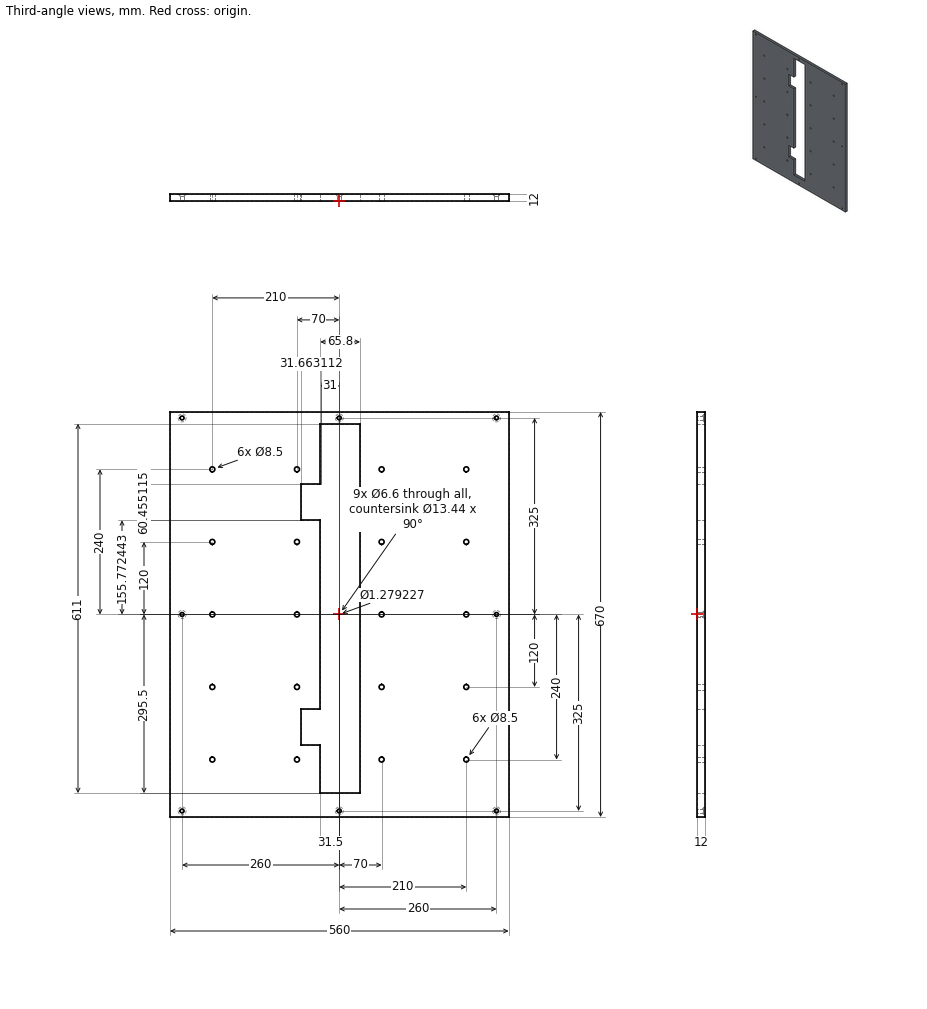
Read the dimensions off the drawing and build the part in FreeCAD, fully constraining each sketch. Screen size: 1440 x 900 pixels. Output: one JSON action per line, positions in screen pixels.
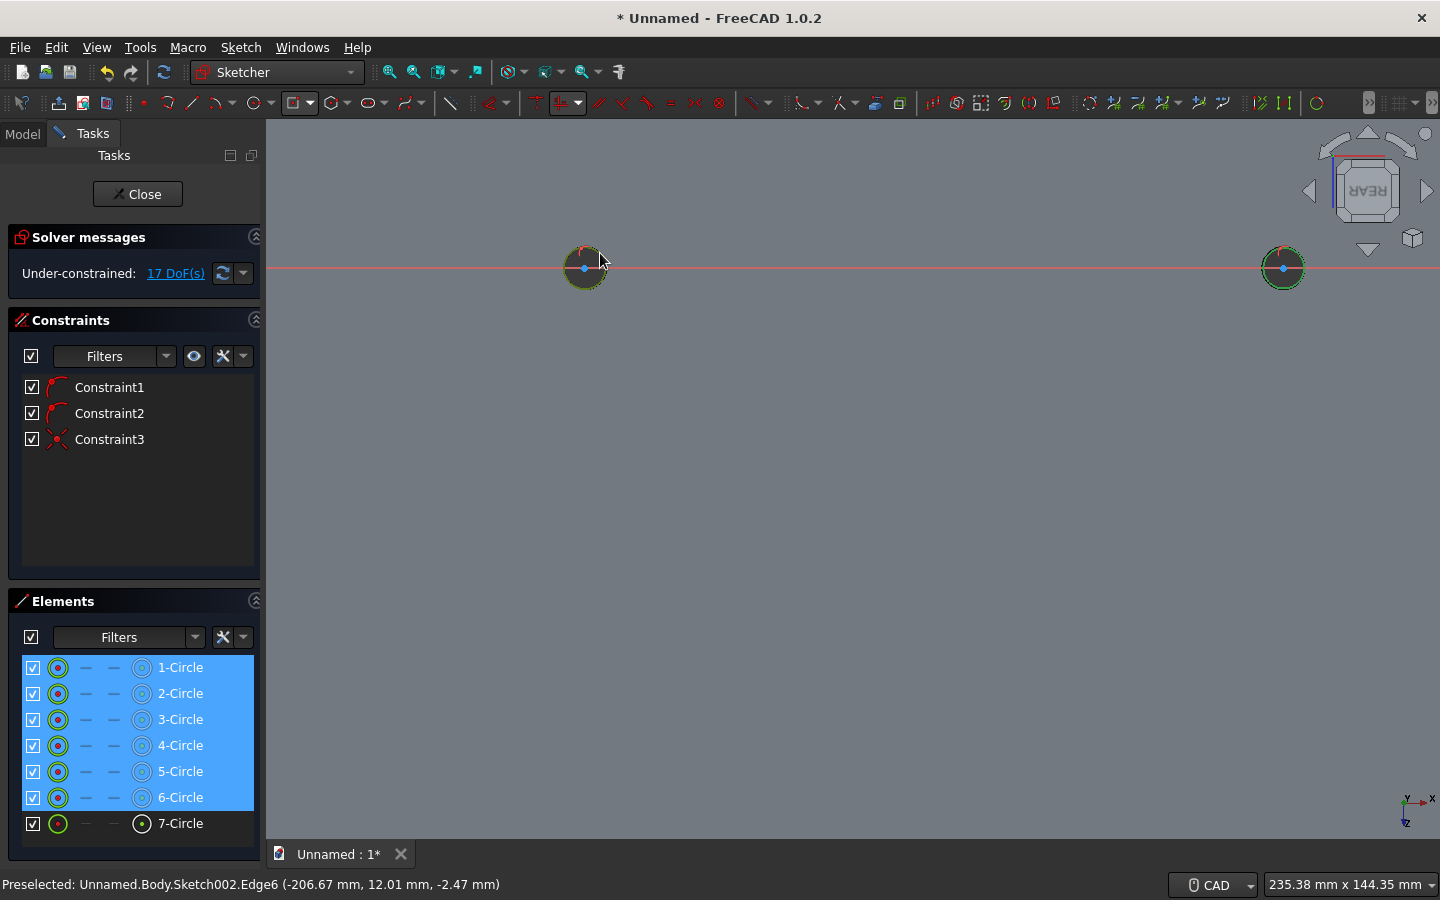
{"action": "left_click", "coordinate": [672, 104]}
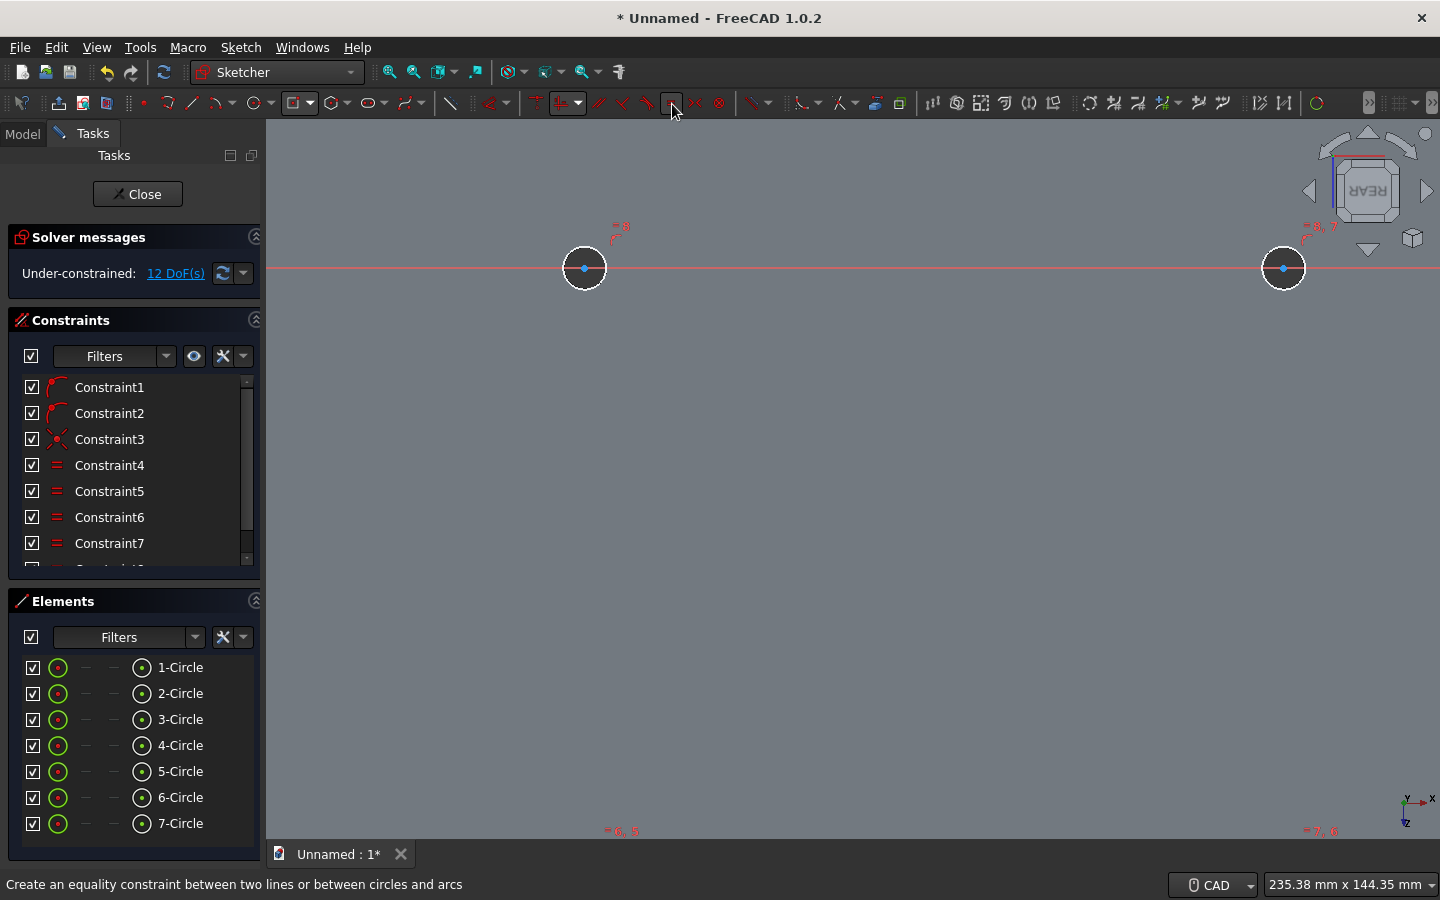
{"action": "scroll", "coordinate": [601, 253], "scroll_direction": "down", "scroll_amount": 5}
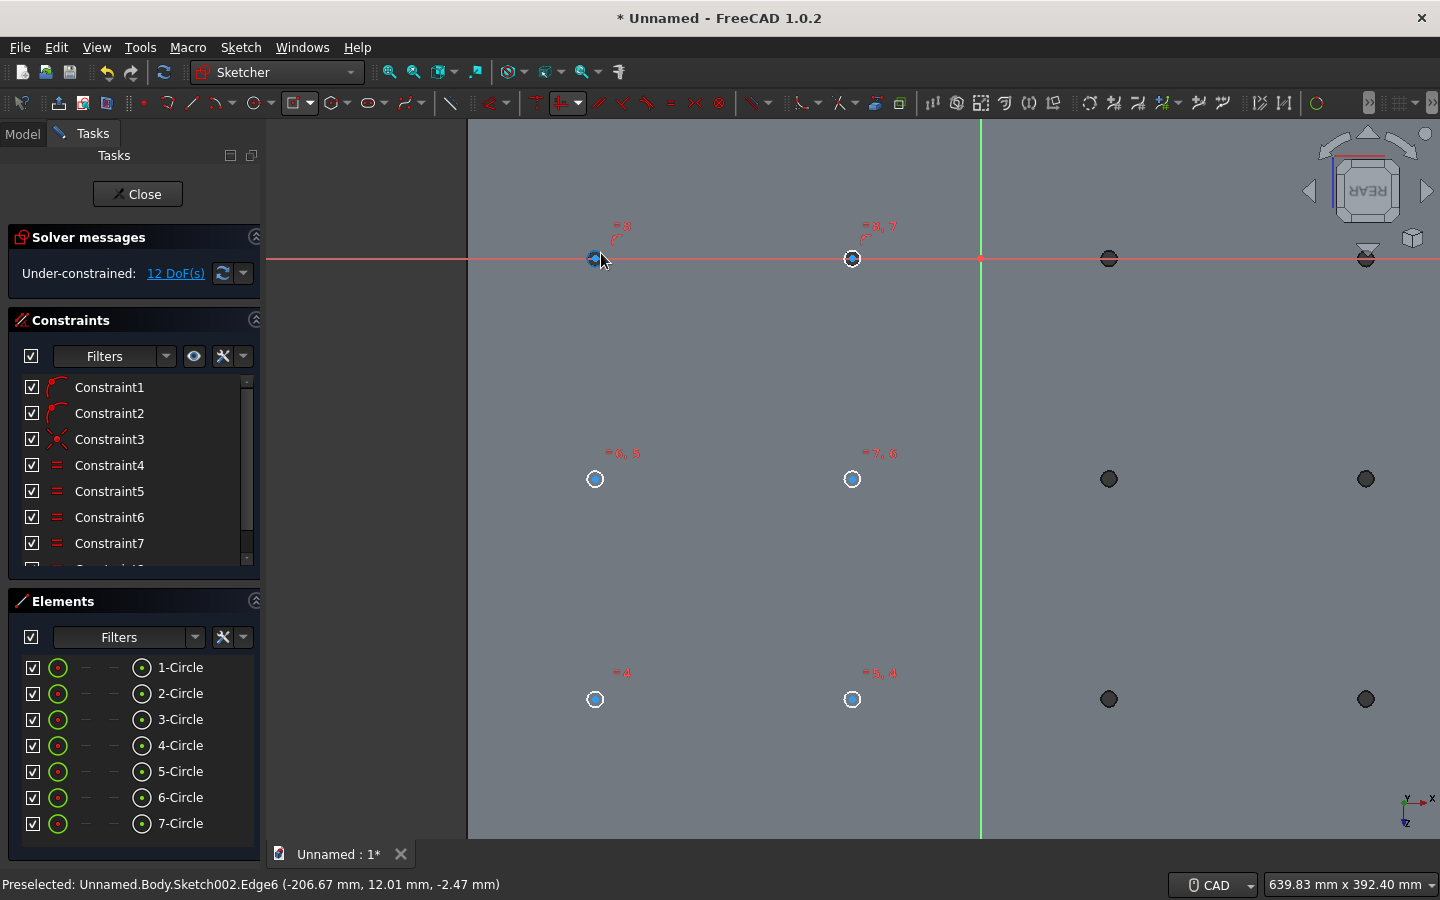
{"action": "left_click", "coordinate": [595, 699]}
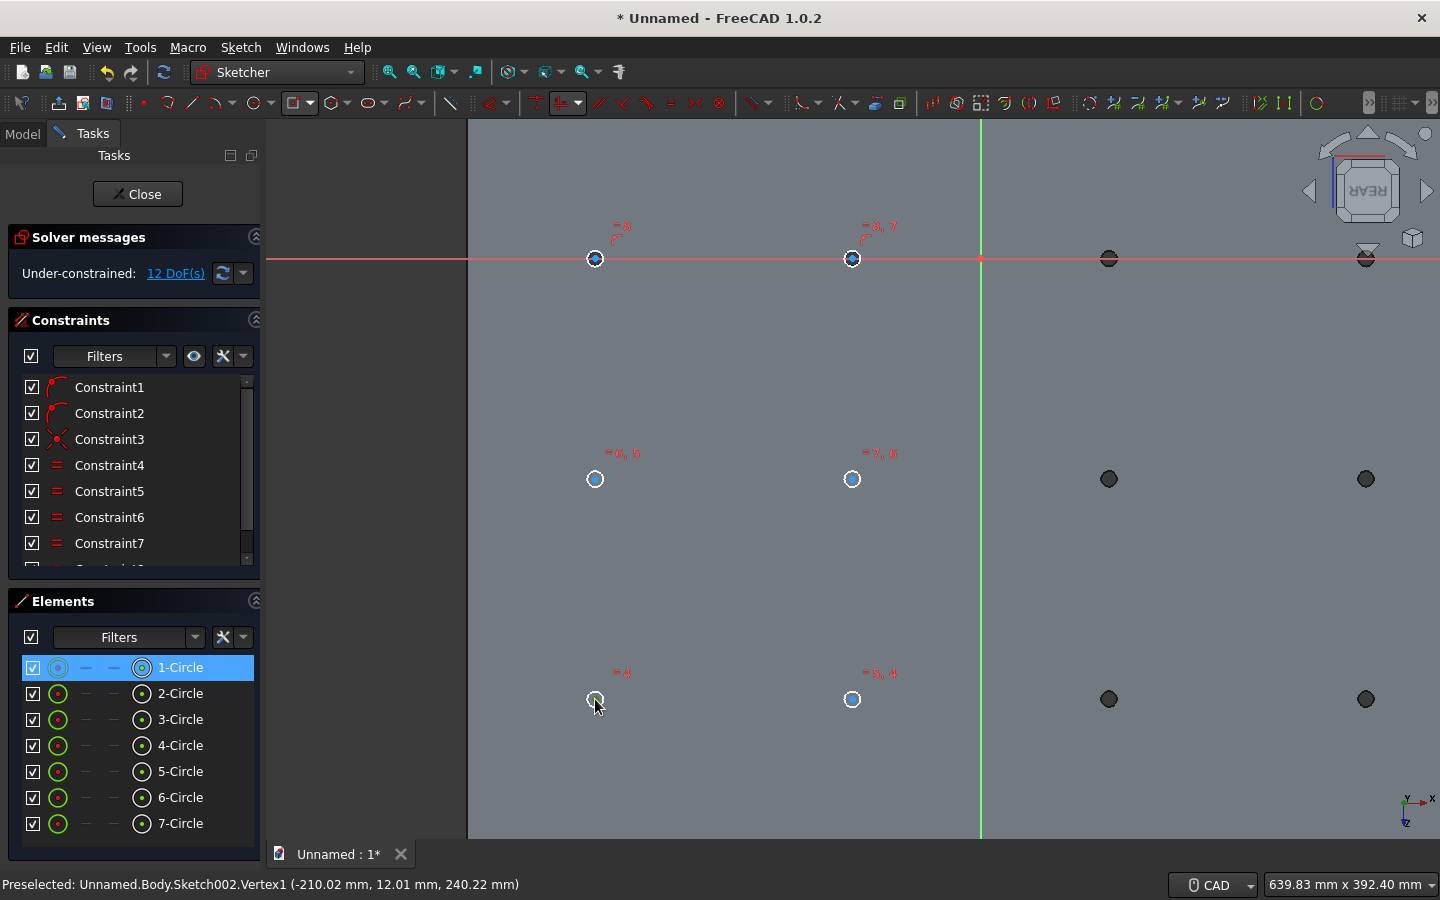
{"action": "left_click", "coordinate": [852, 699]}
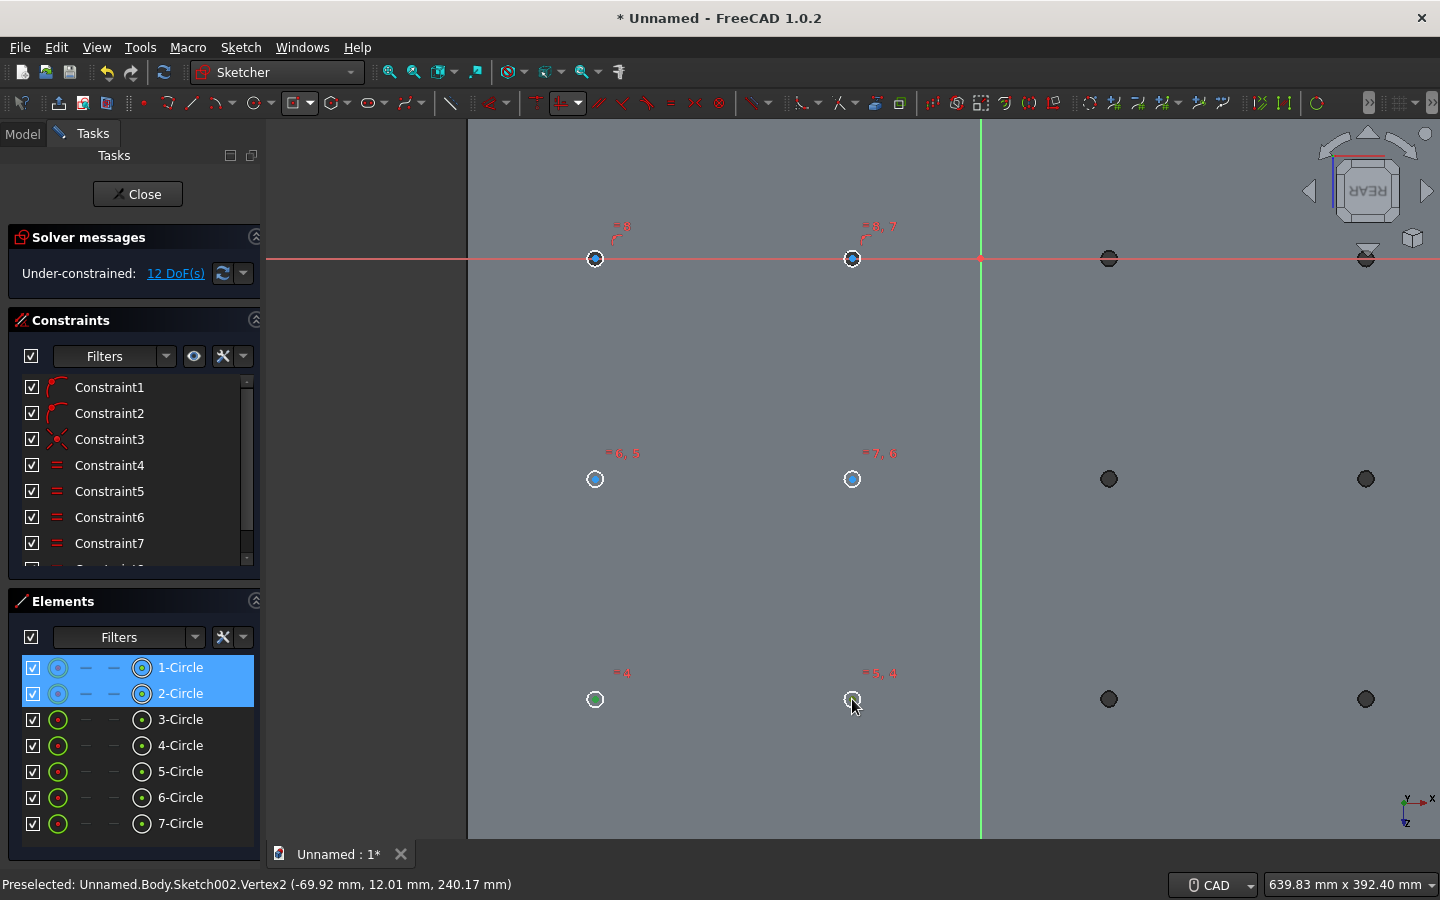
{"action": "left_click", "coordinate": [580, 104]}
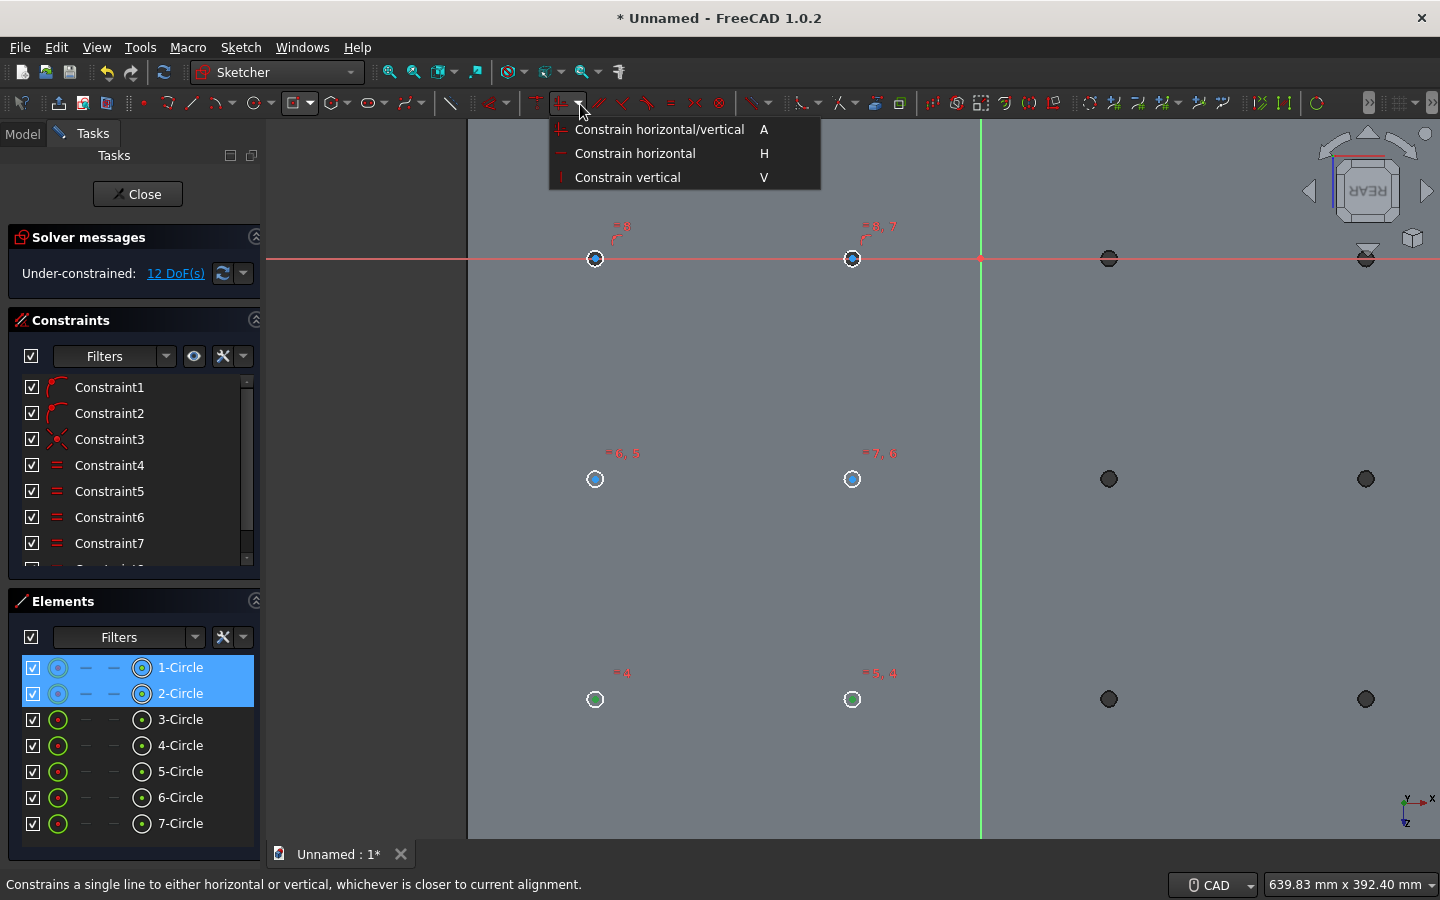
{"action": "left_click", "coordinate": [685, 153]}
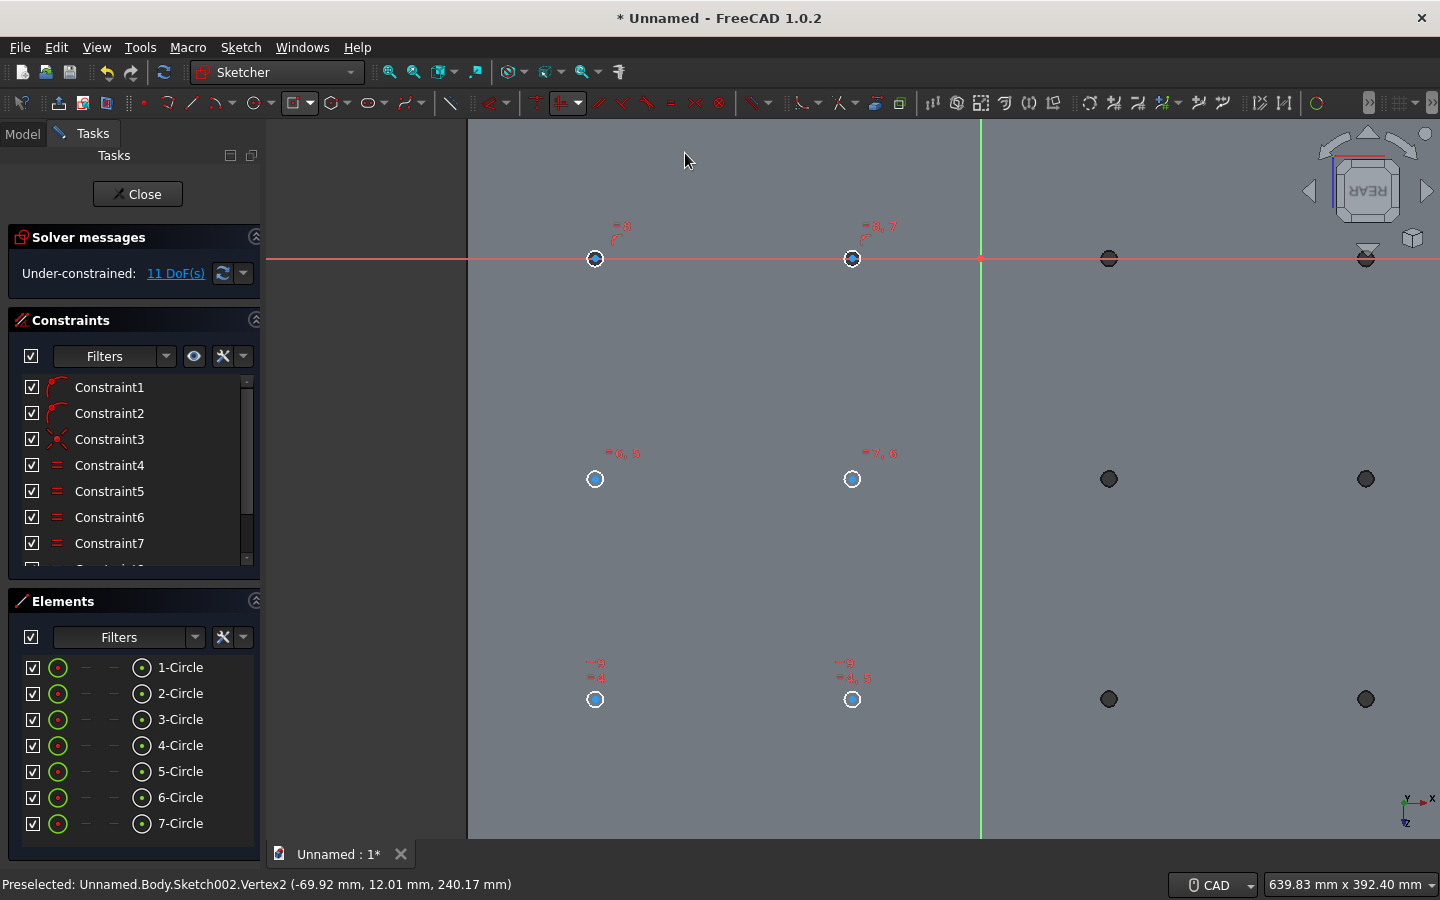
{"action": "left_click", "coordinate": [595, 699]}